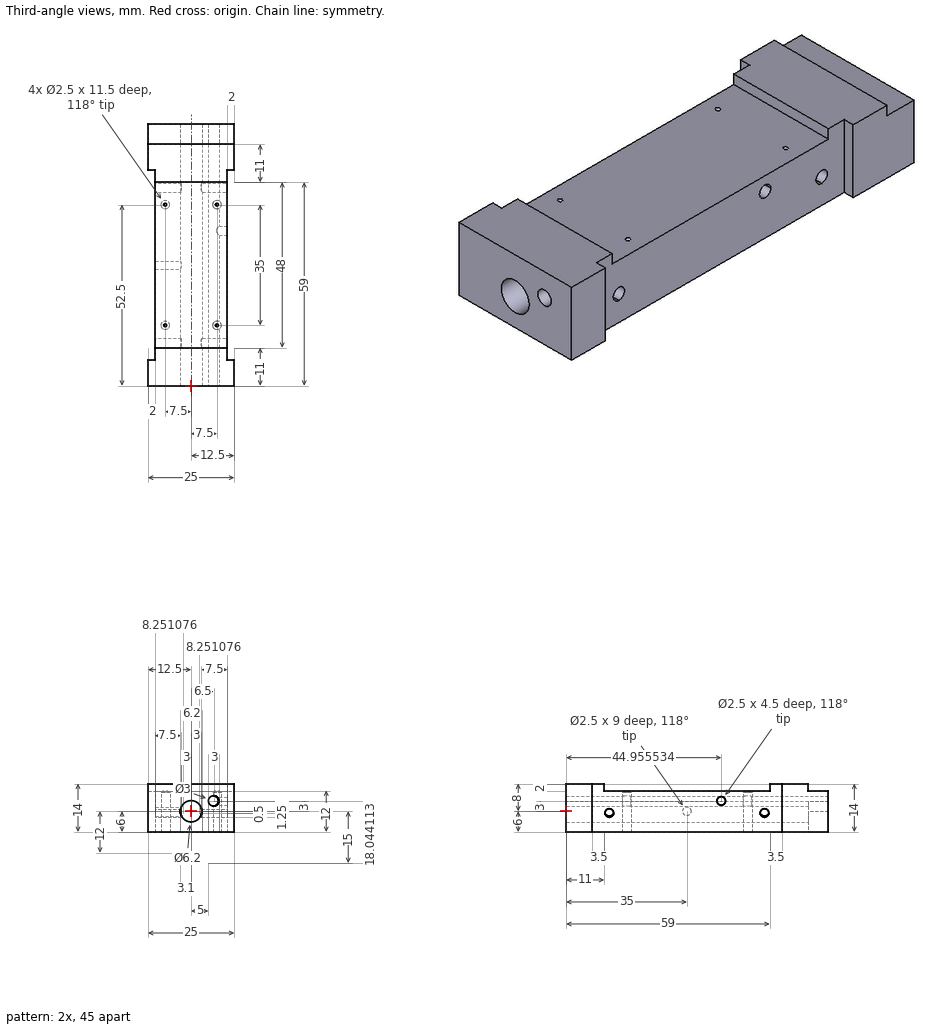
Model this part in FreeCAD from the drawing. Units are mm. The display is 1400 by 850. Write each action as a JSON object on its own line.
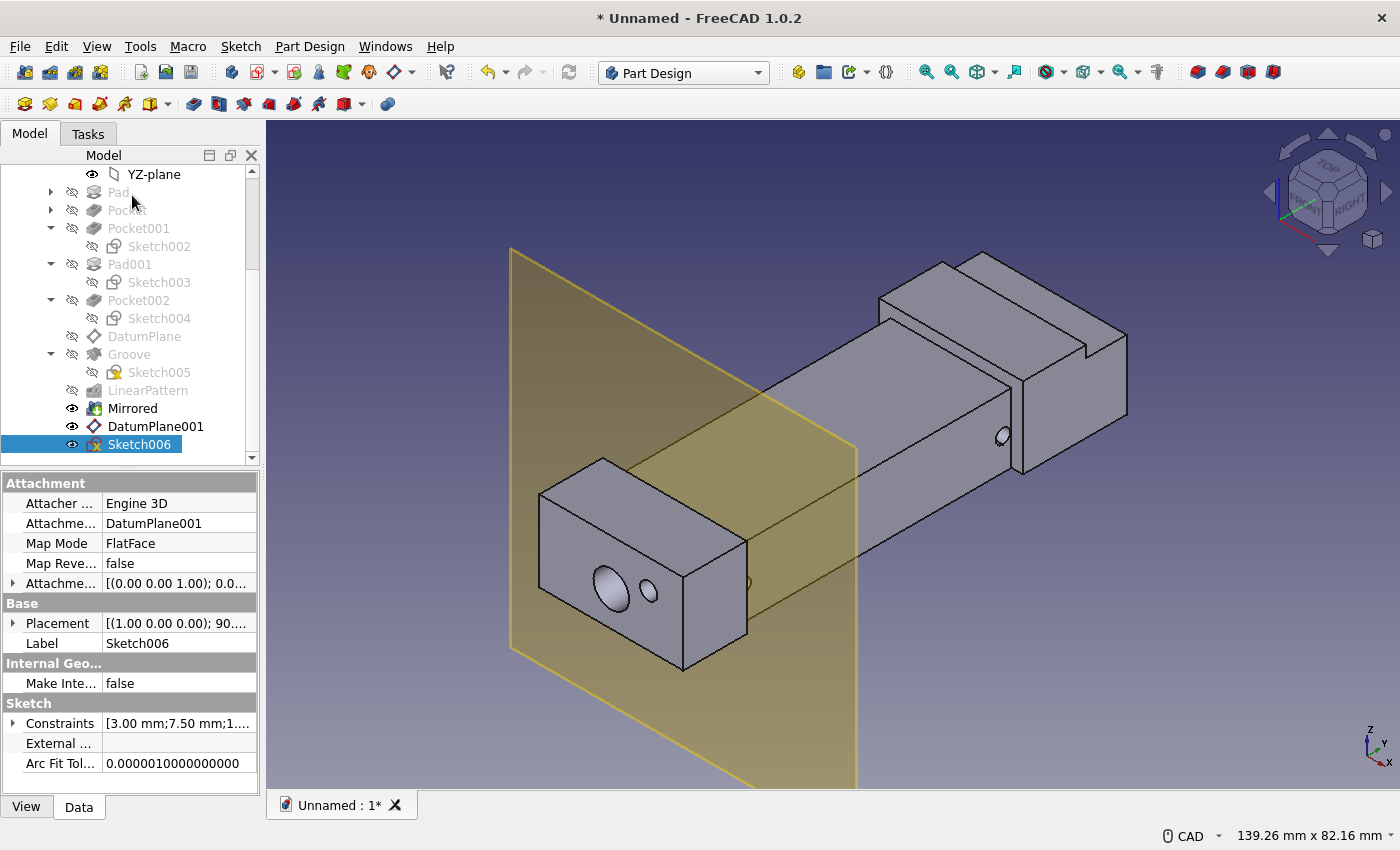
{"action": "left_click", "coordinate": [244, 104]}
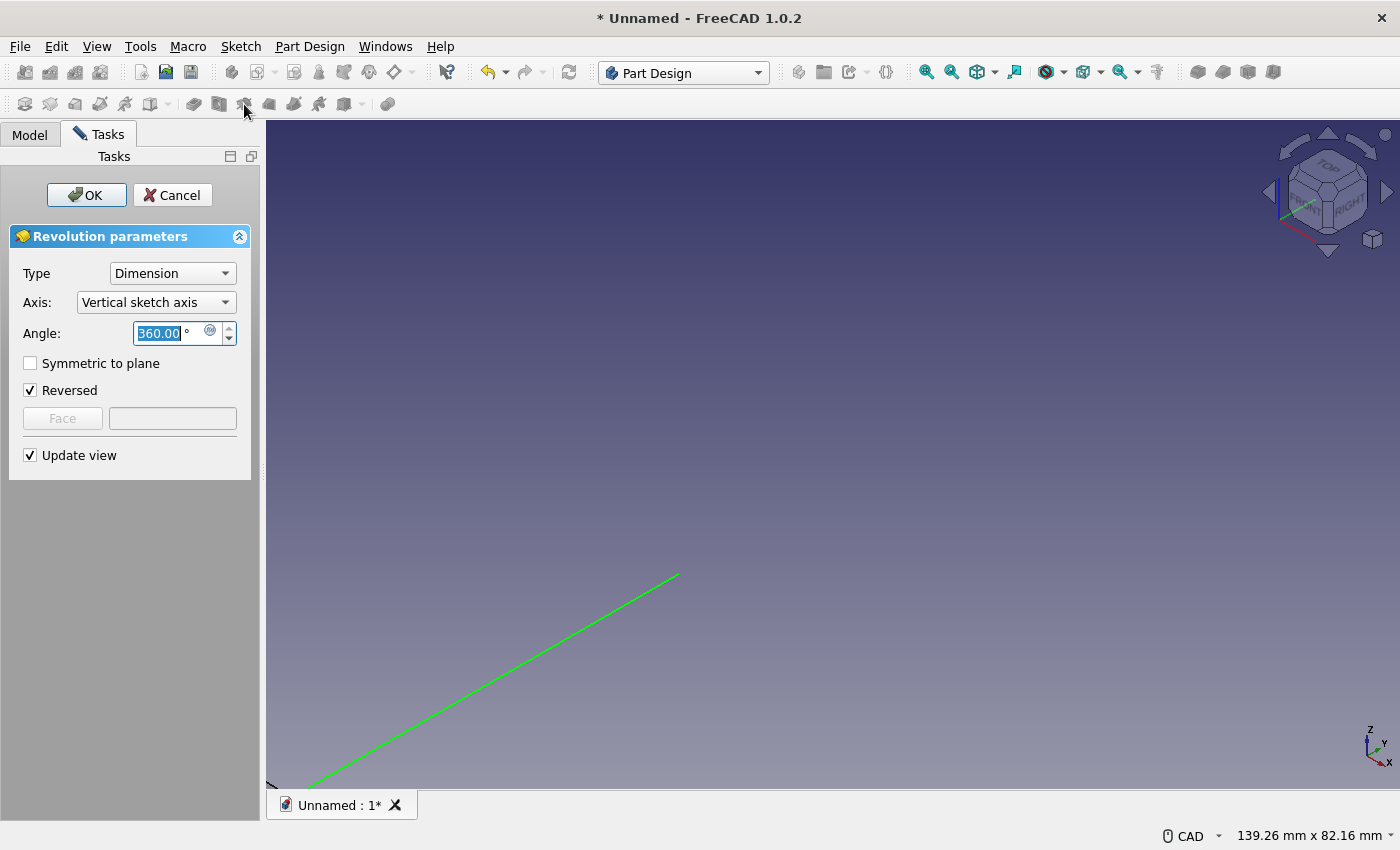
{"action": "left_click", "coordinate": [157, 302]}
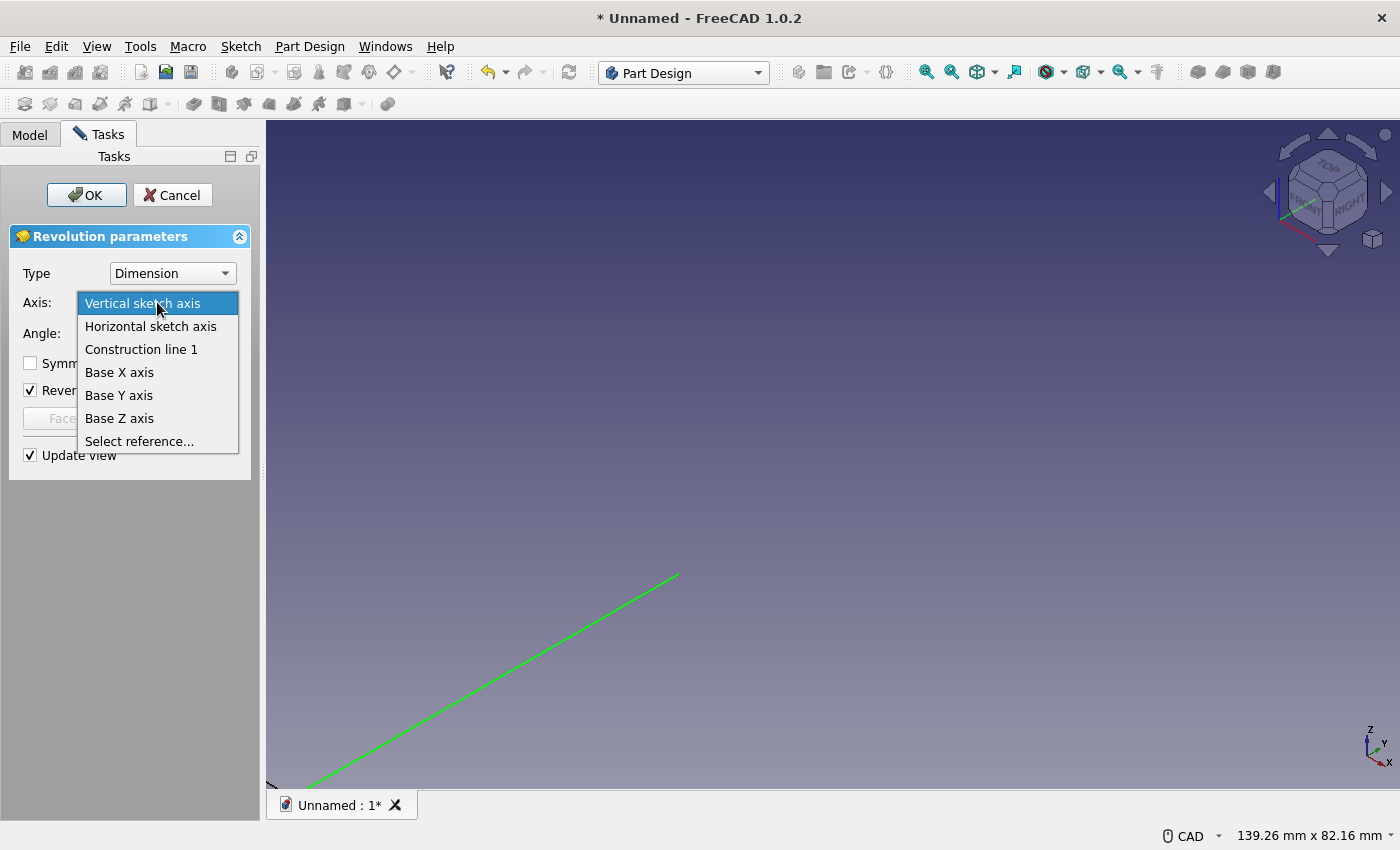
{"action": "left_click", "coordinate": [156, 350]}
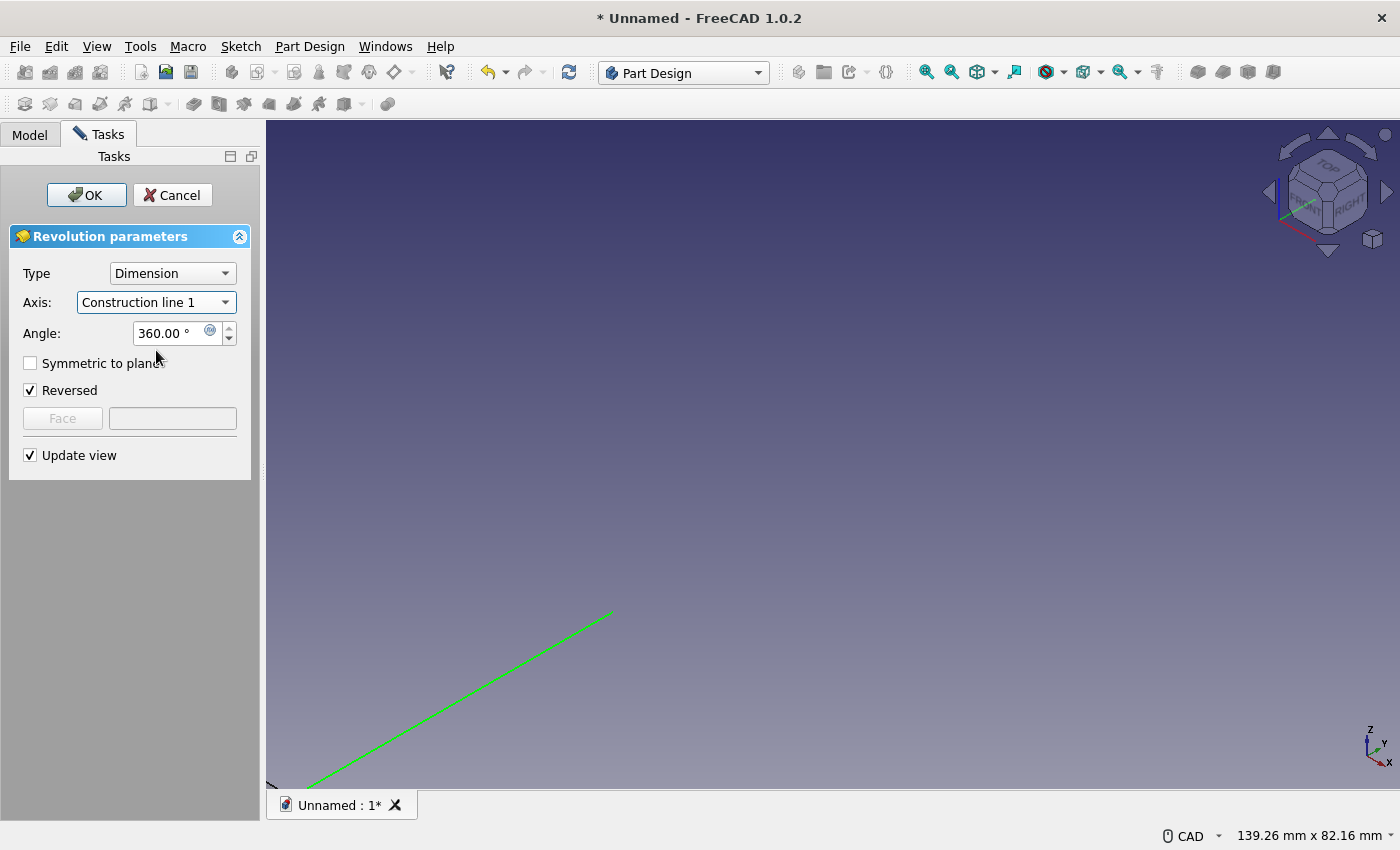
{"action": "left_click", "coordinate": [87, 195]}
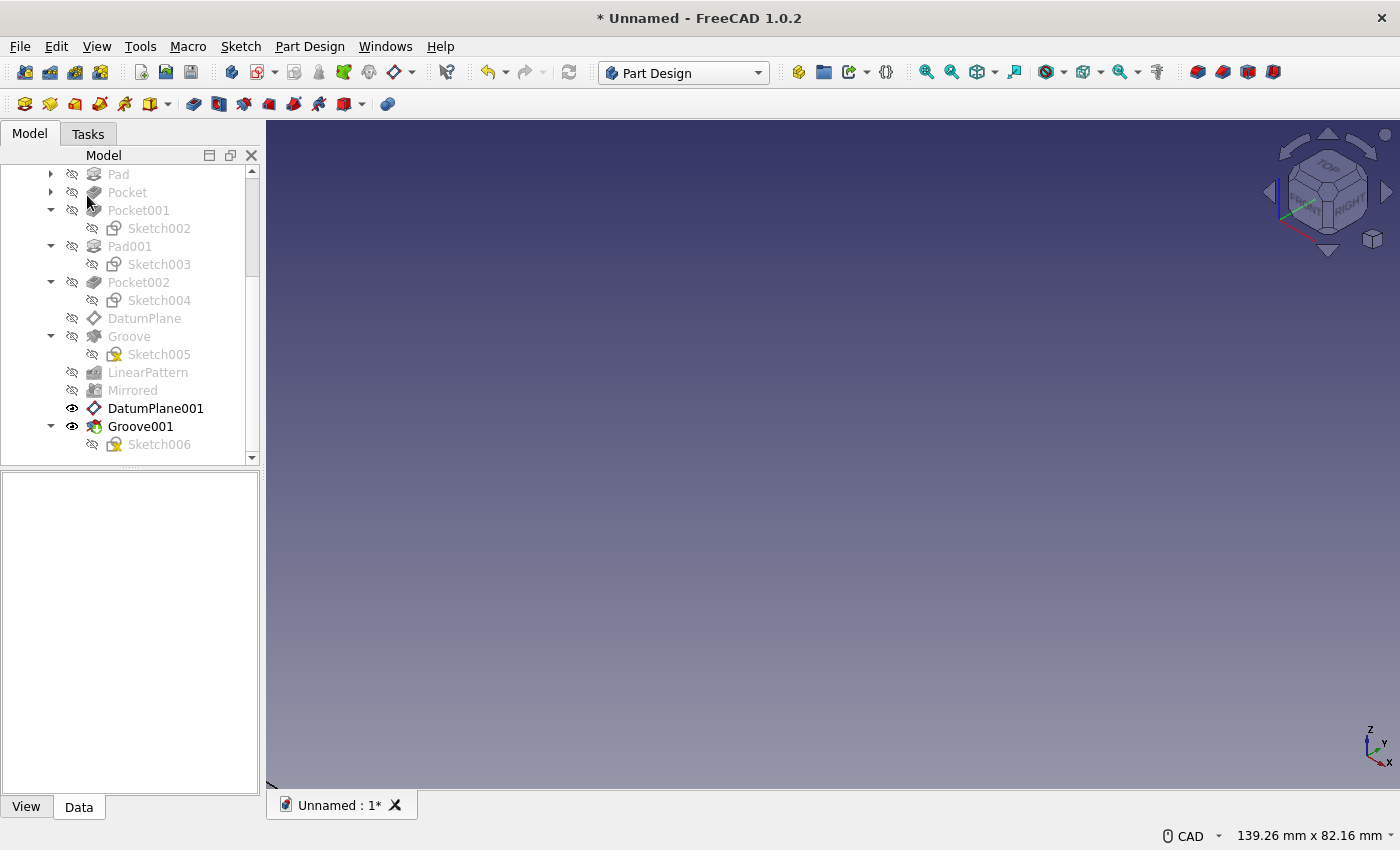
{"action": "left_click", "coordinate": [117, 408]}
{"action": "key", "text": "space"}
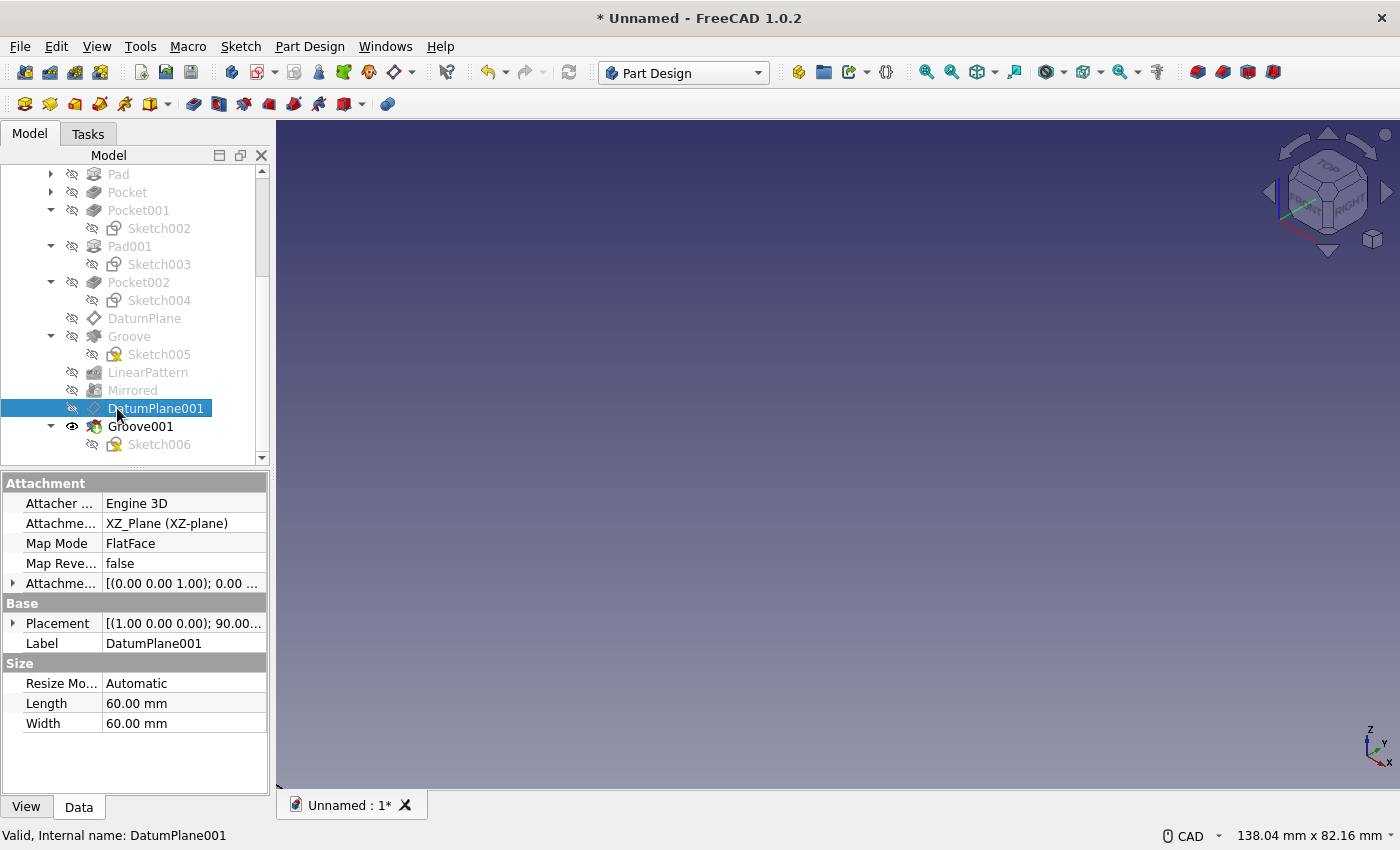
{"action": "left_click", "coordinate": [927, 72]}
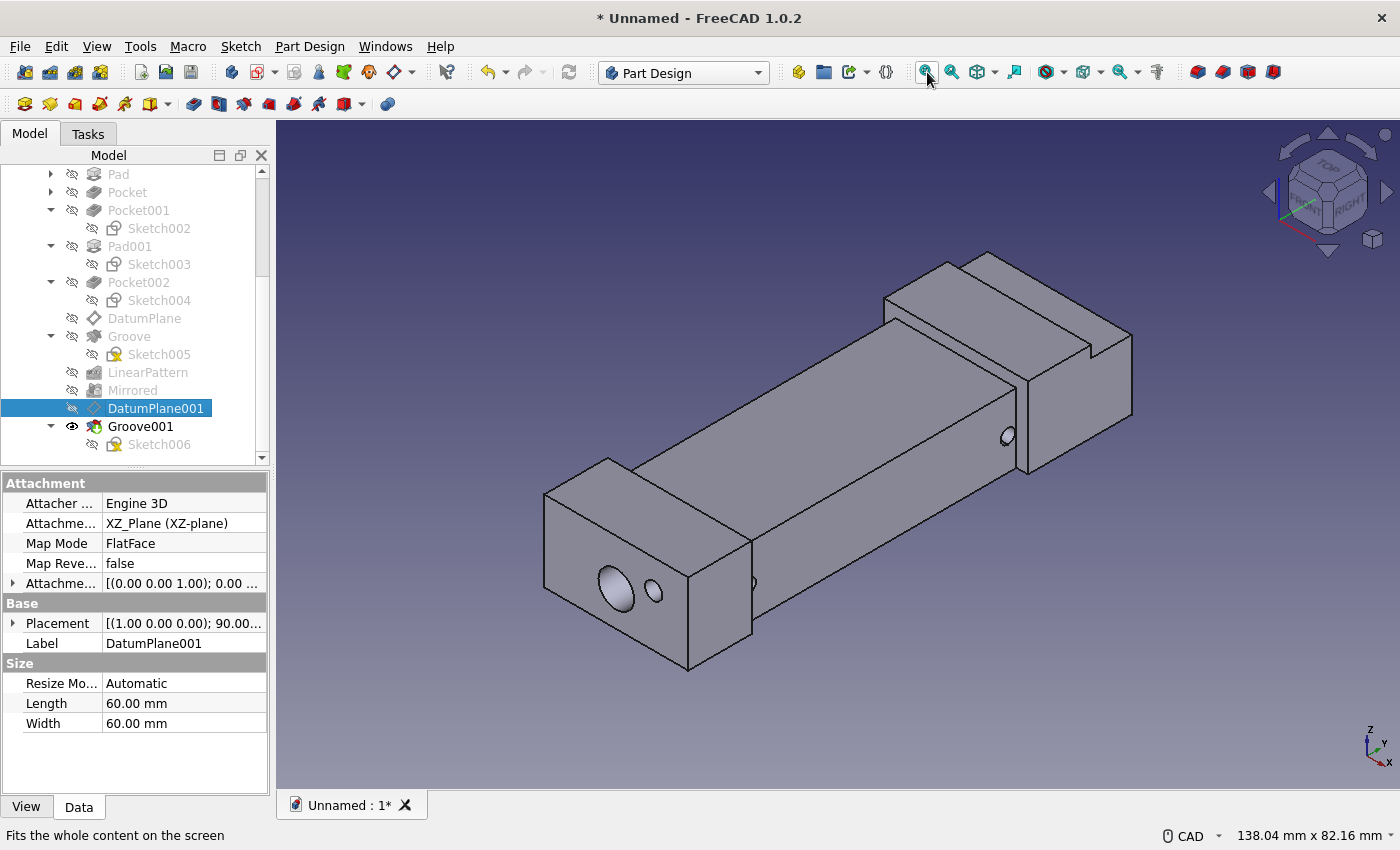
{"action": "key", "text": "5"}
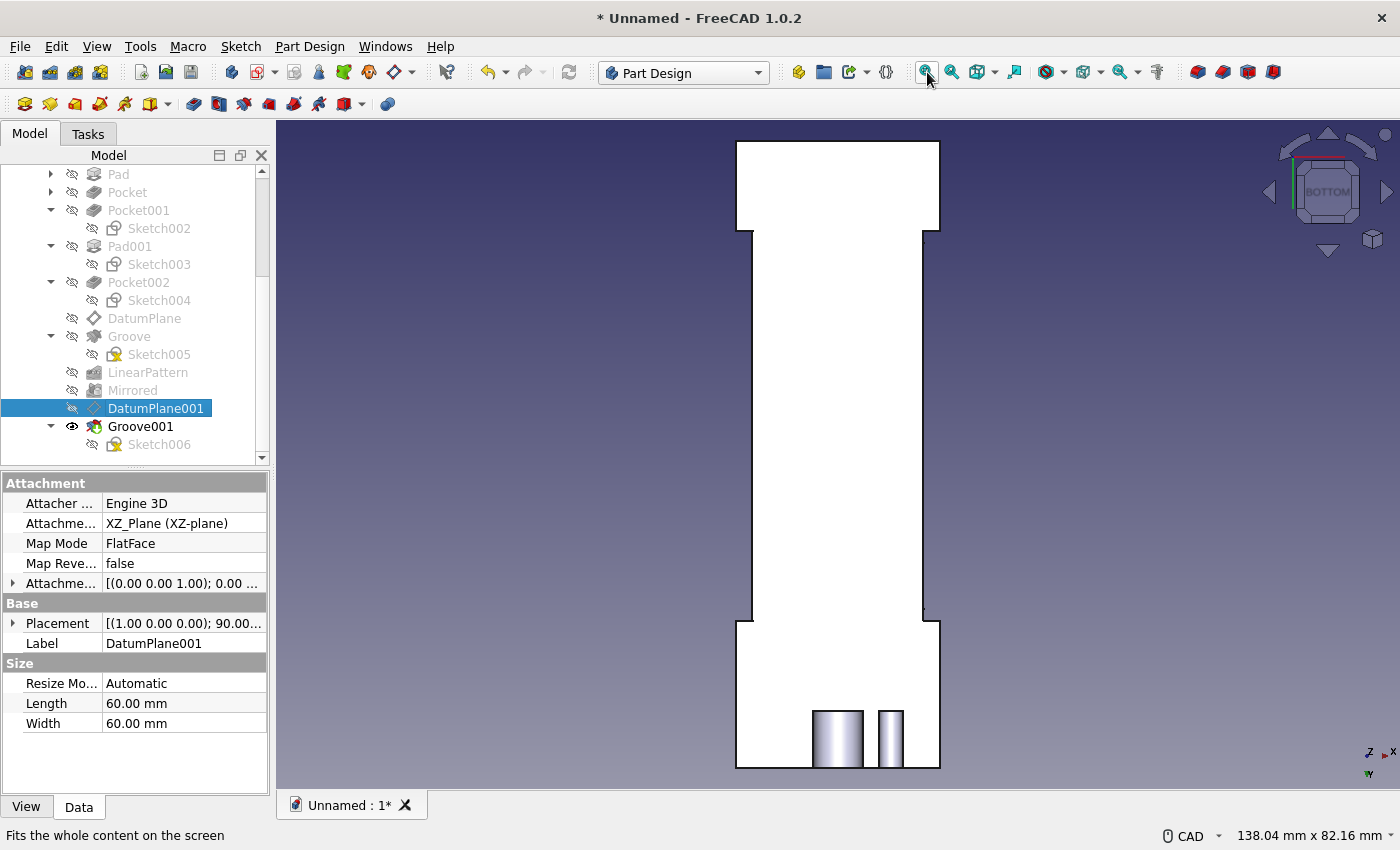
{"action": "left_click", "coordinate": [838, 543]}